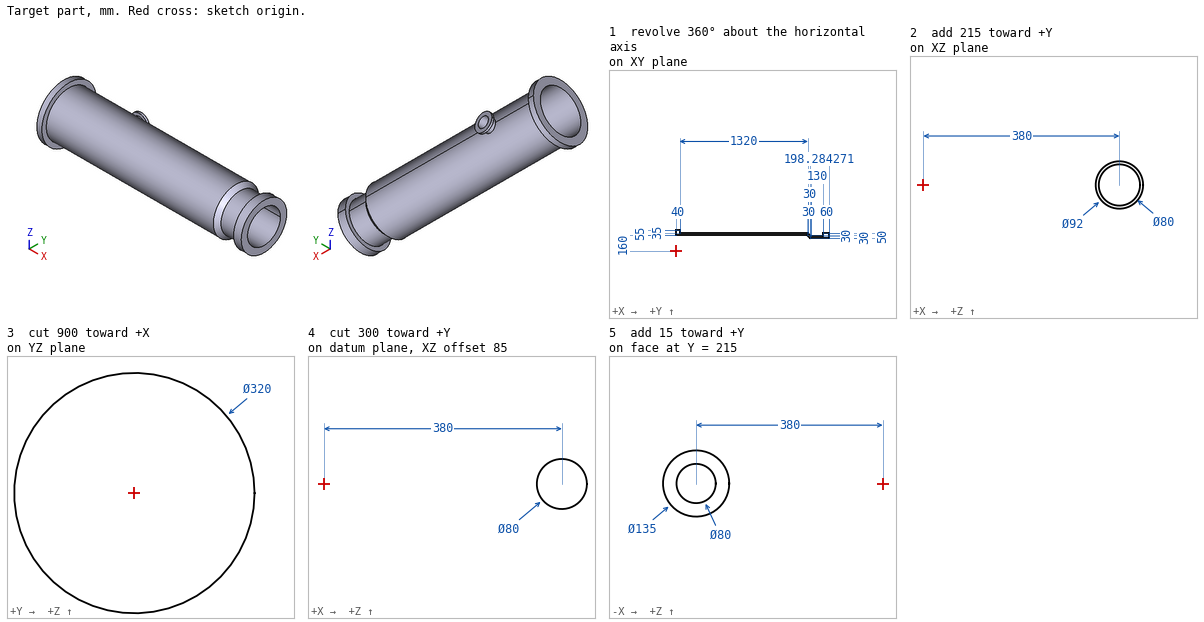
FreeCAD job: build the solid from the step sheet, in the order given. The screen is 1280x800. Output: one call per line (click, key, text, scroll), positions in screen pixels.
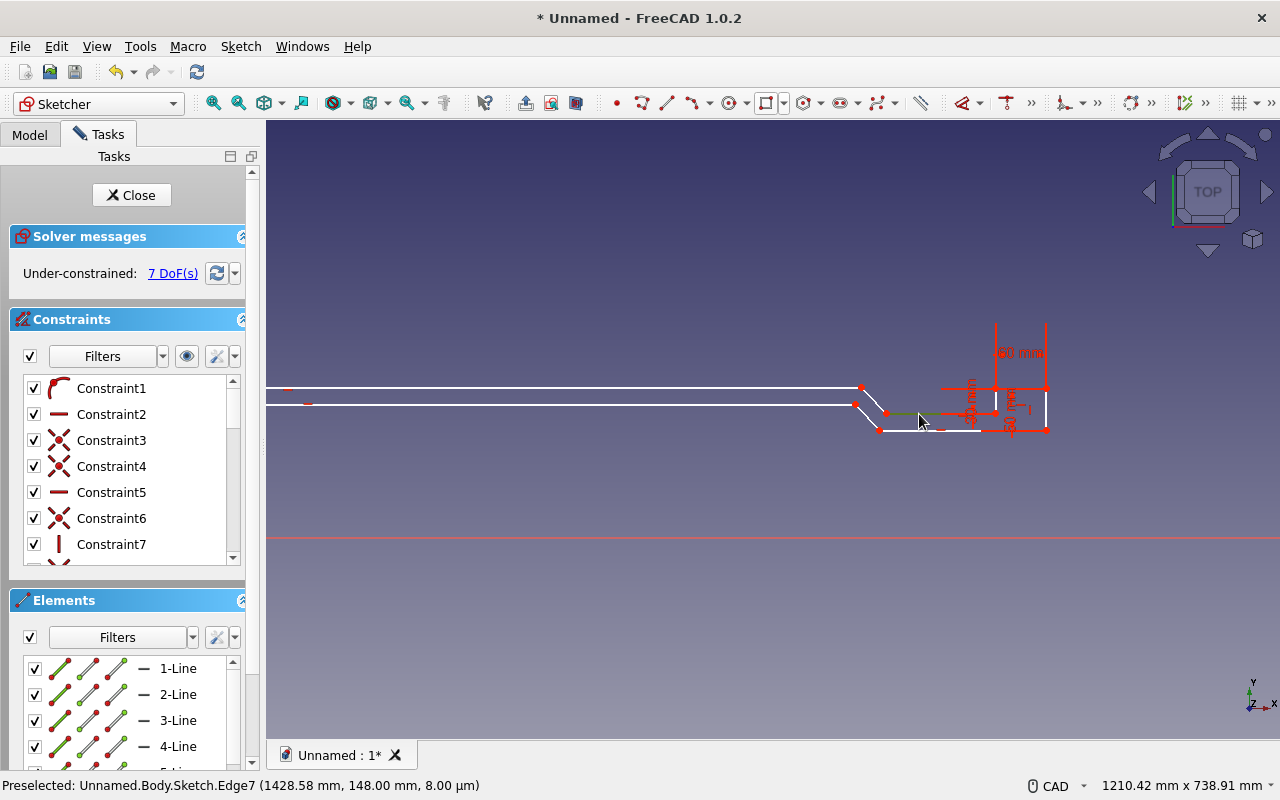
key(l)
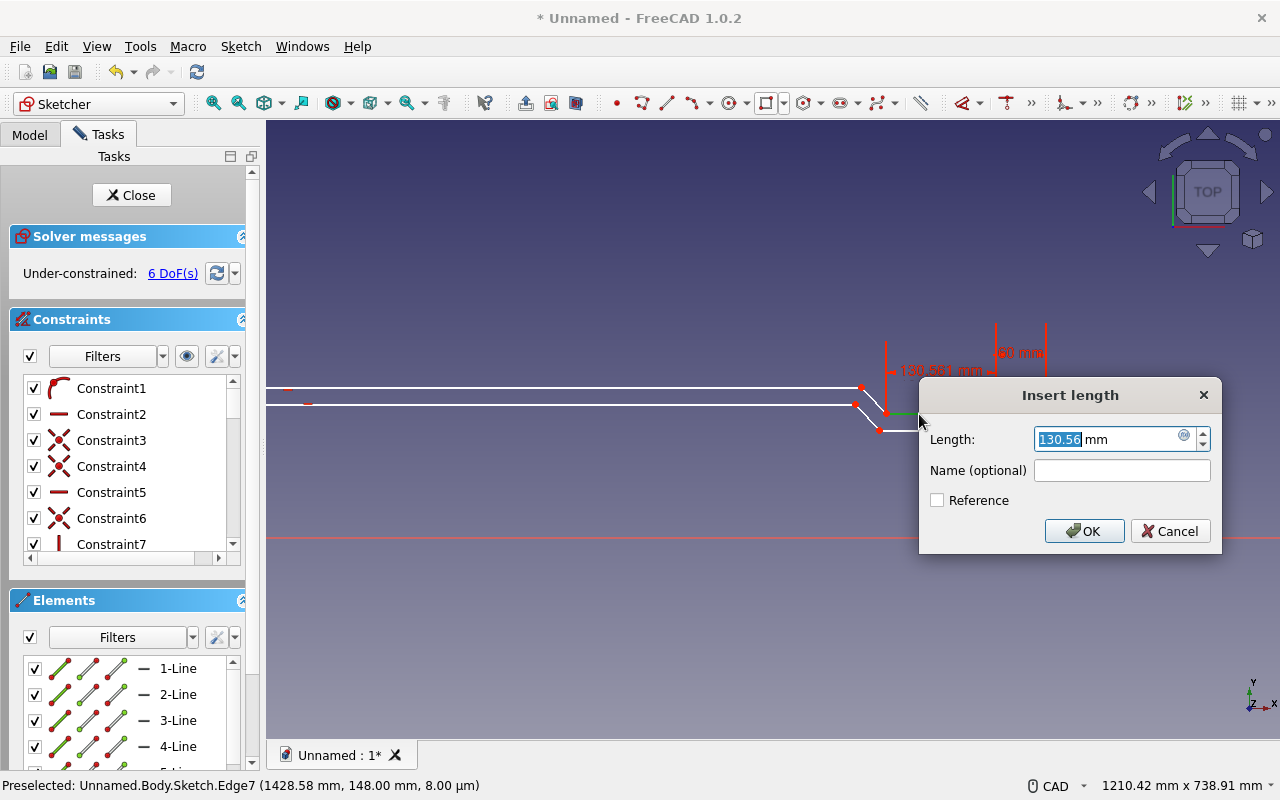
text(130)
key(Return)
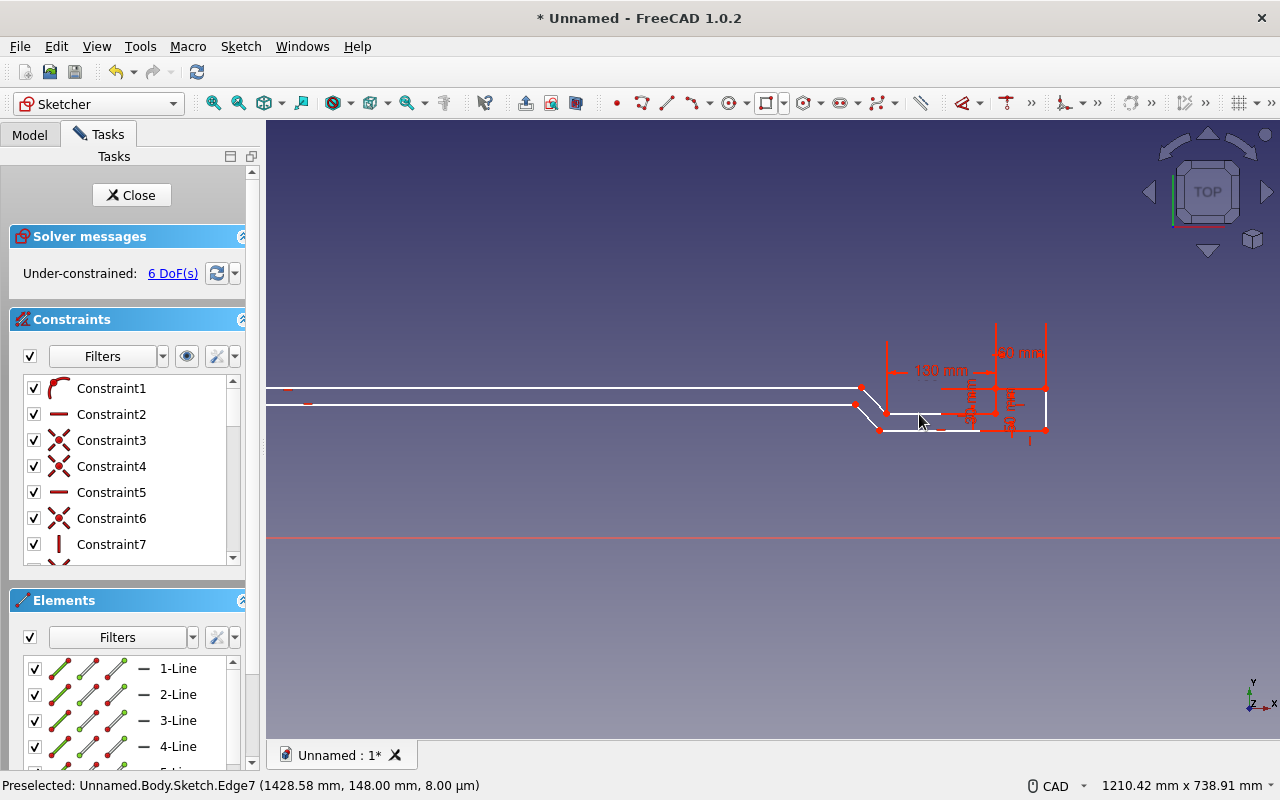
scroll(863, 412, up, 3)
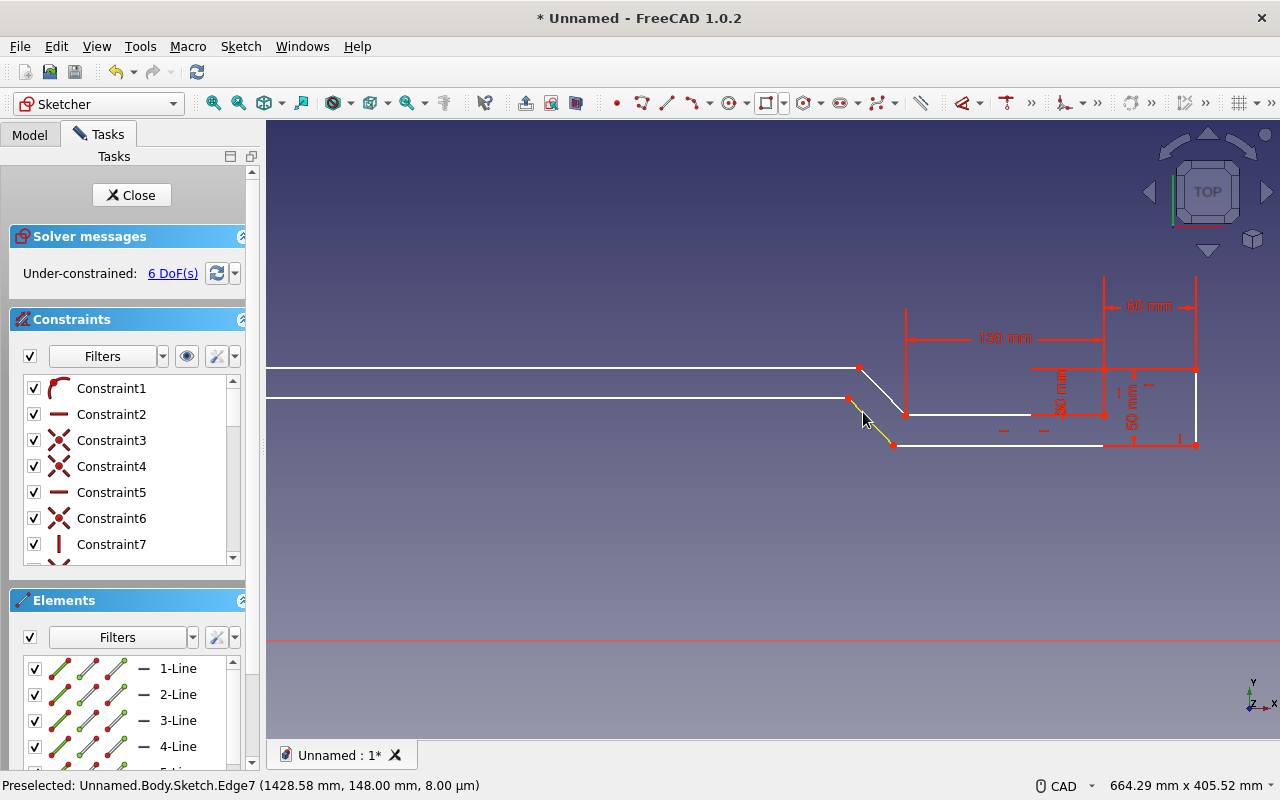
click(862, 412)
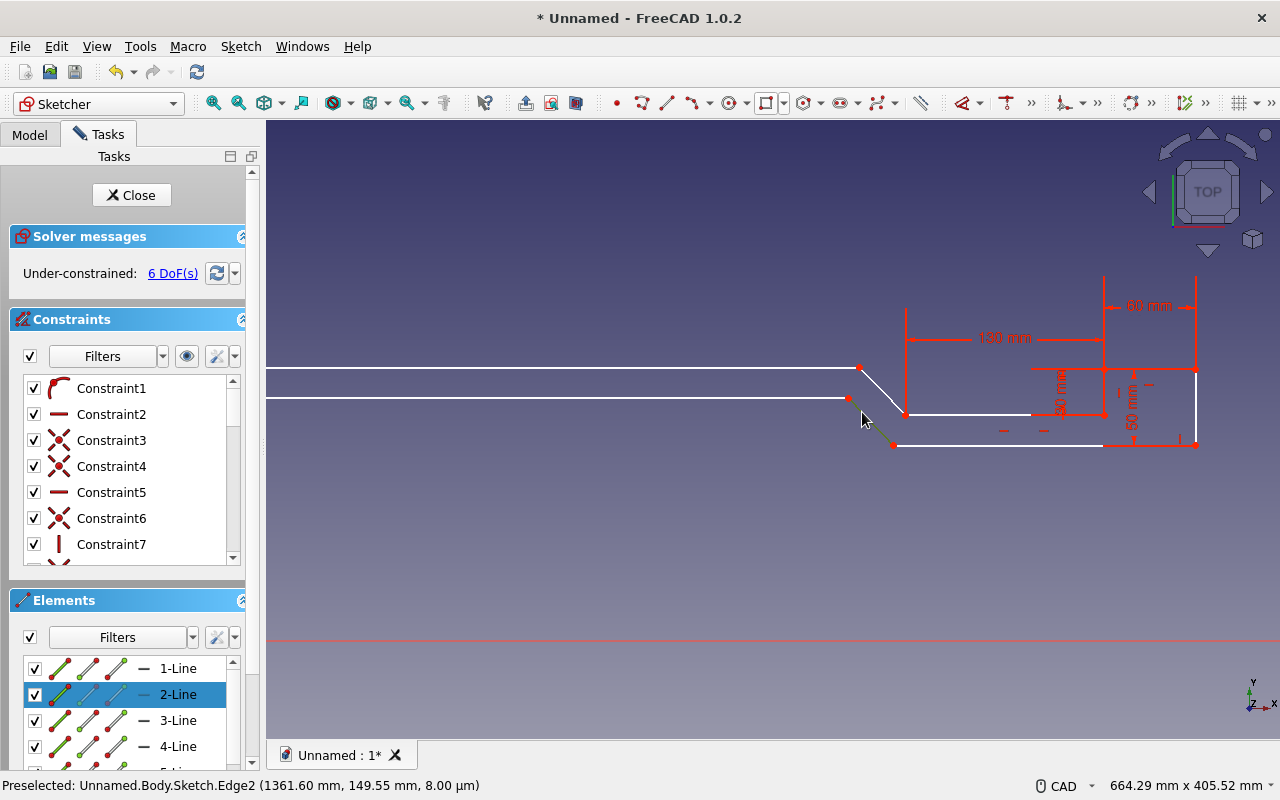
key(l)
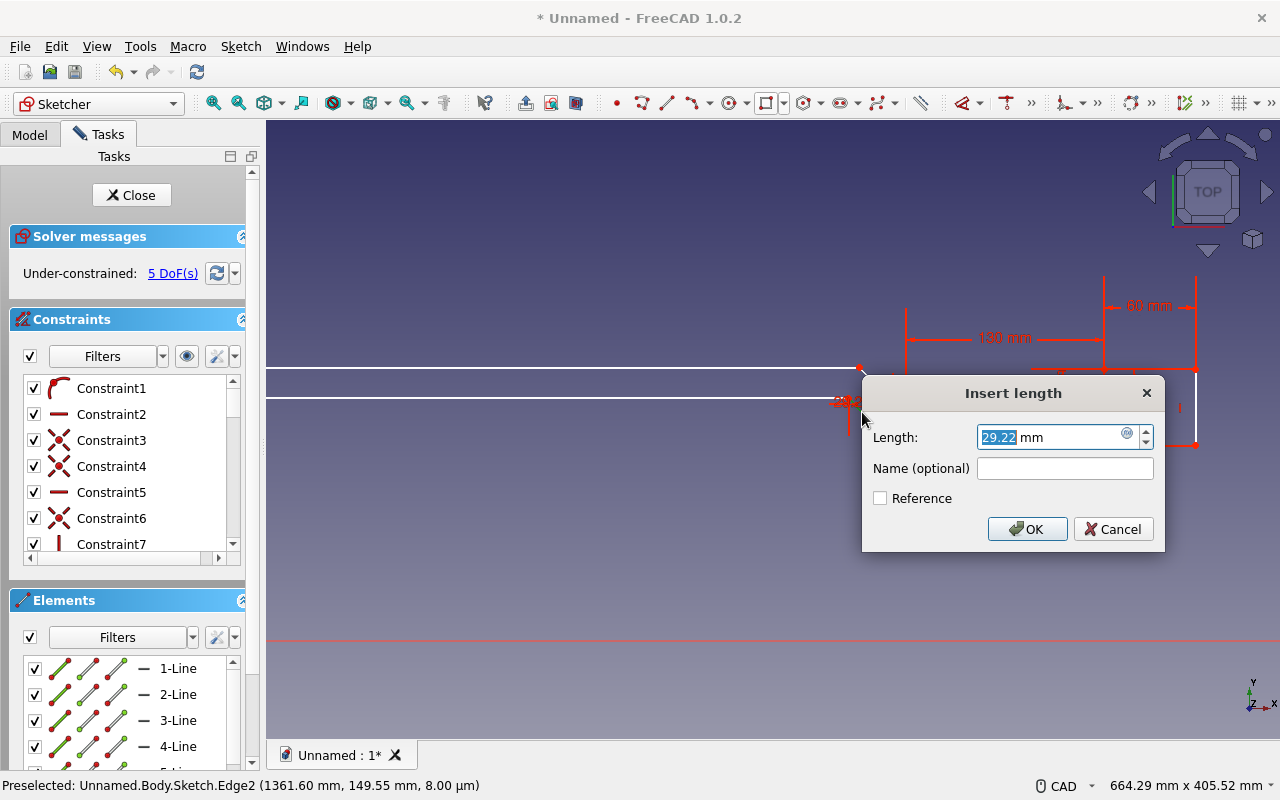
text(30)
key(Return)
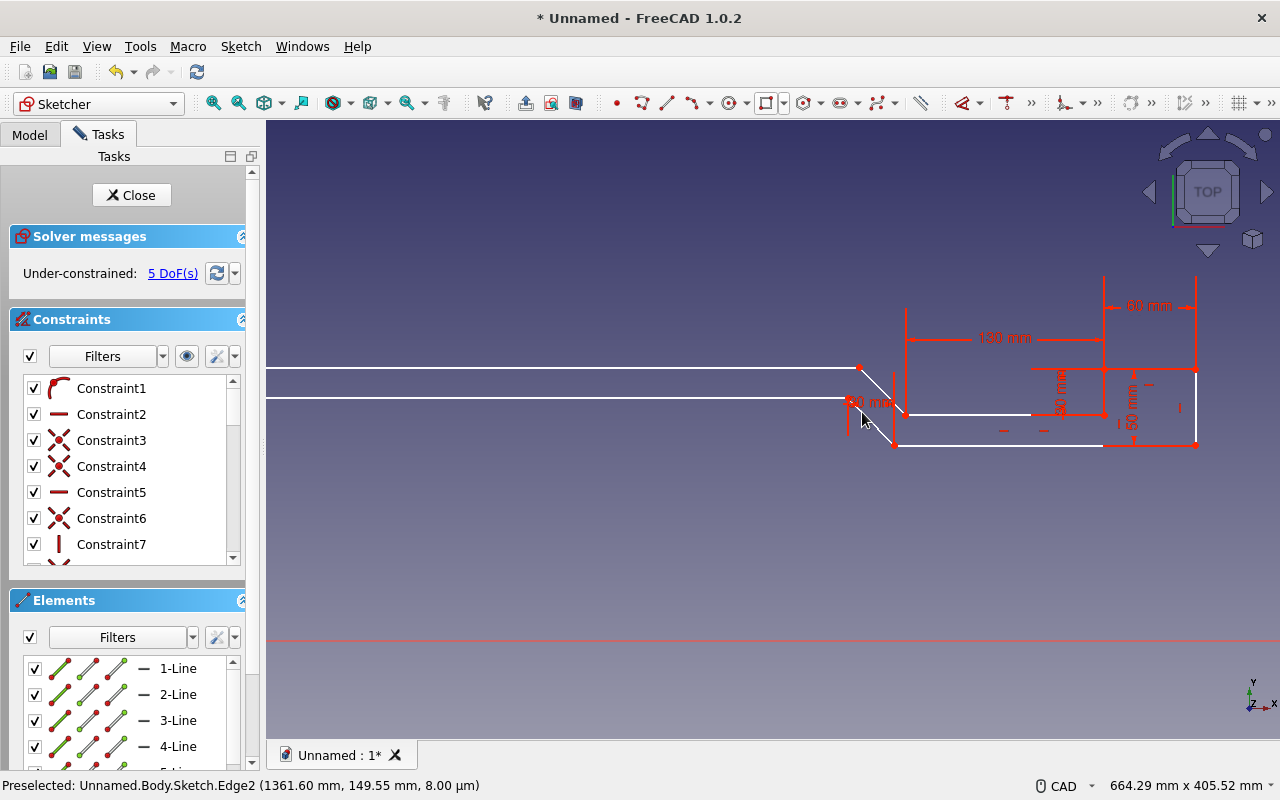
click(862, 412)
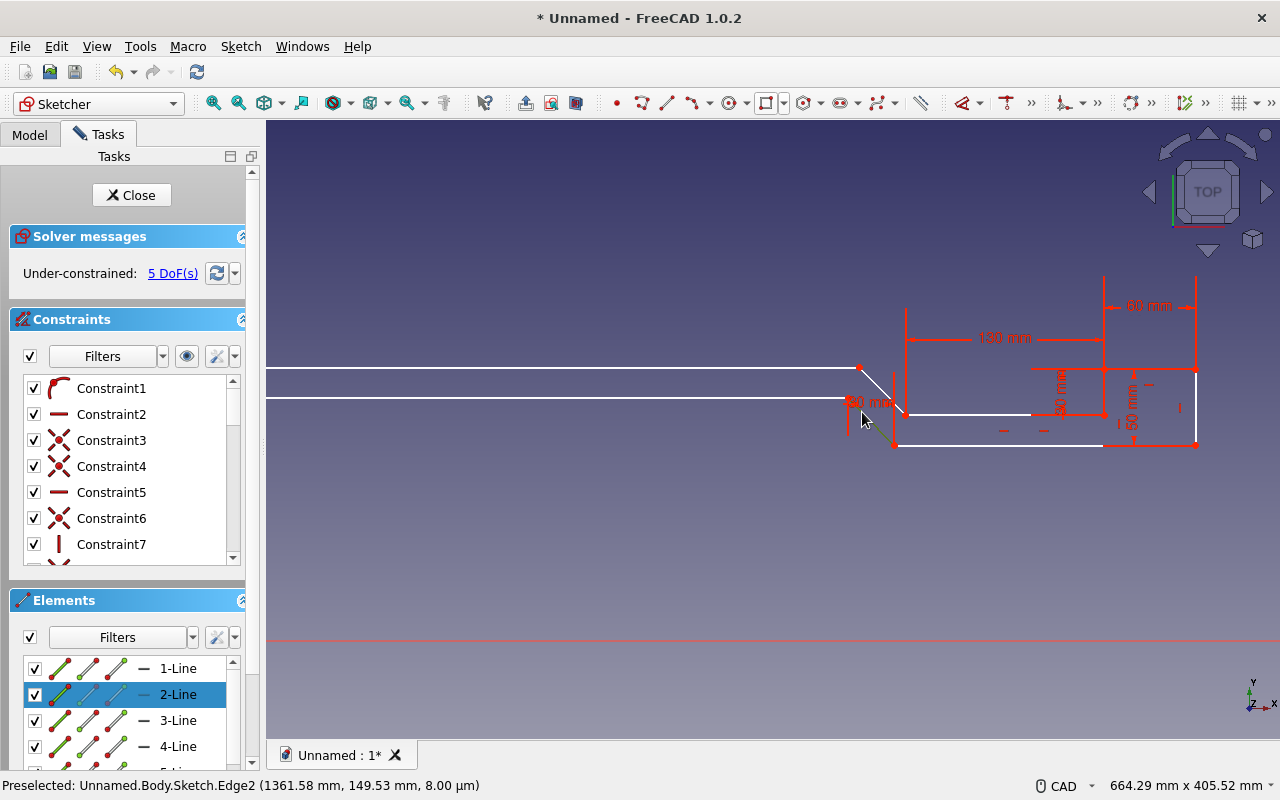
key(i)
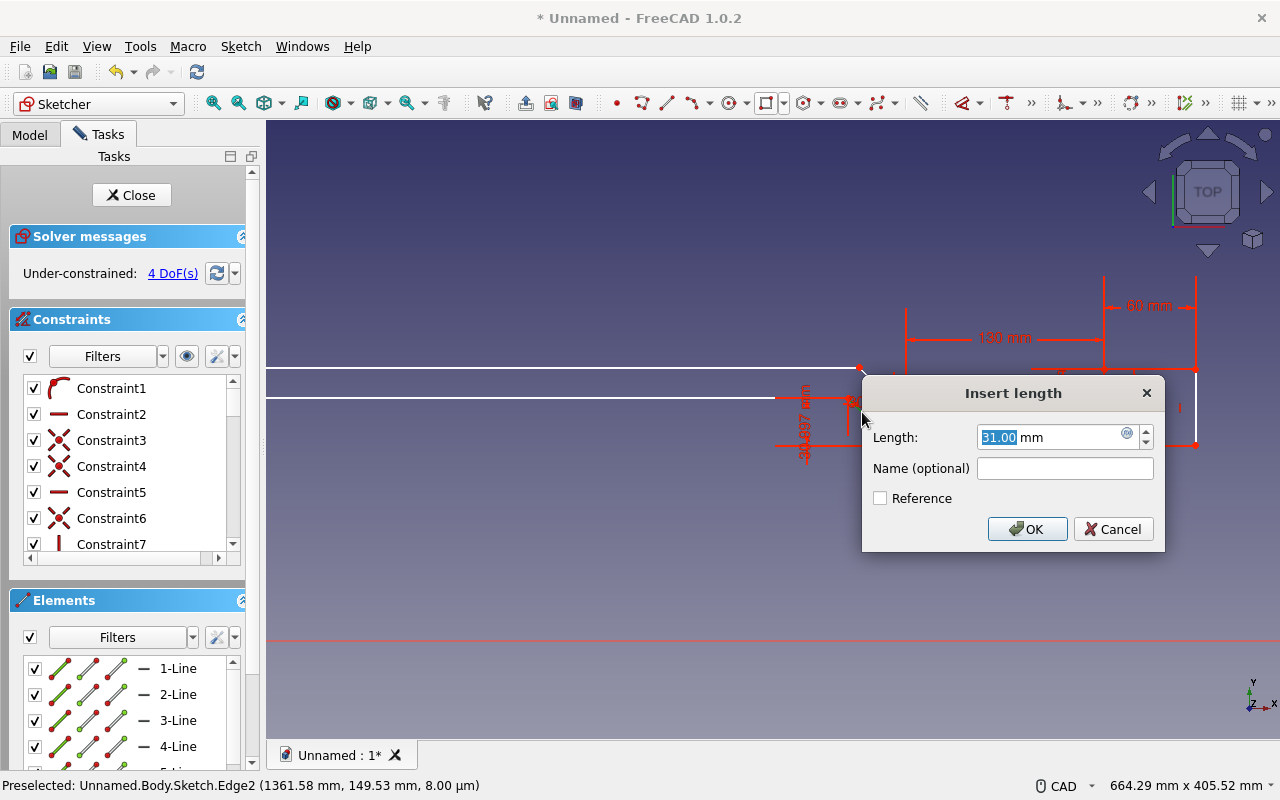
text(30)
key(Return)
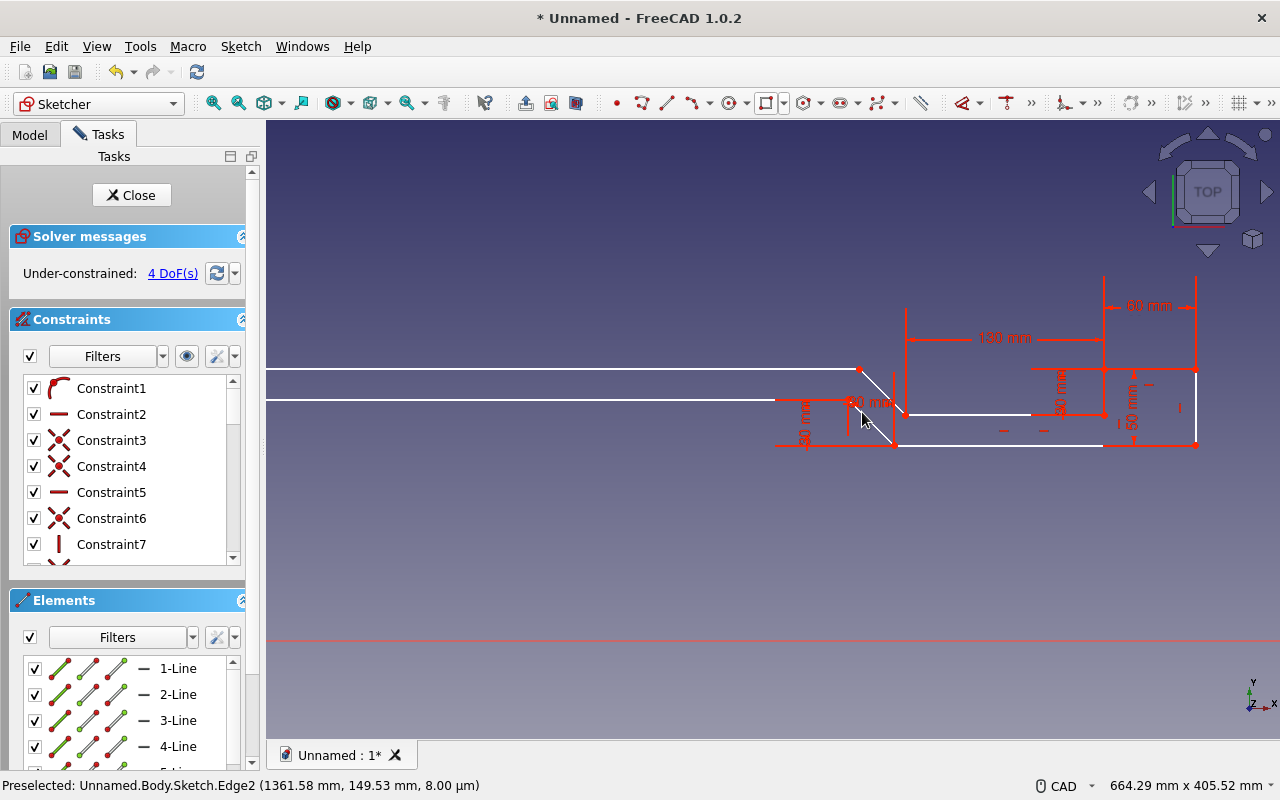
click(874, 383)